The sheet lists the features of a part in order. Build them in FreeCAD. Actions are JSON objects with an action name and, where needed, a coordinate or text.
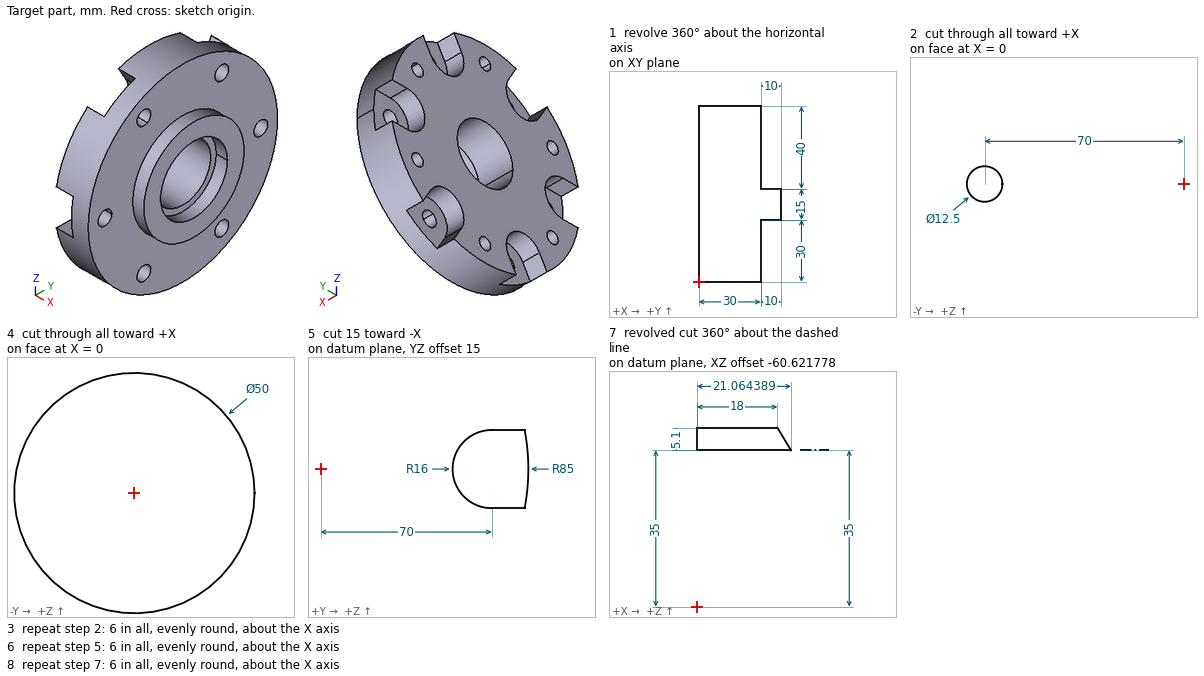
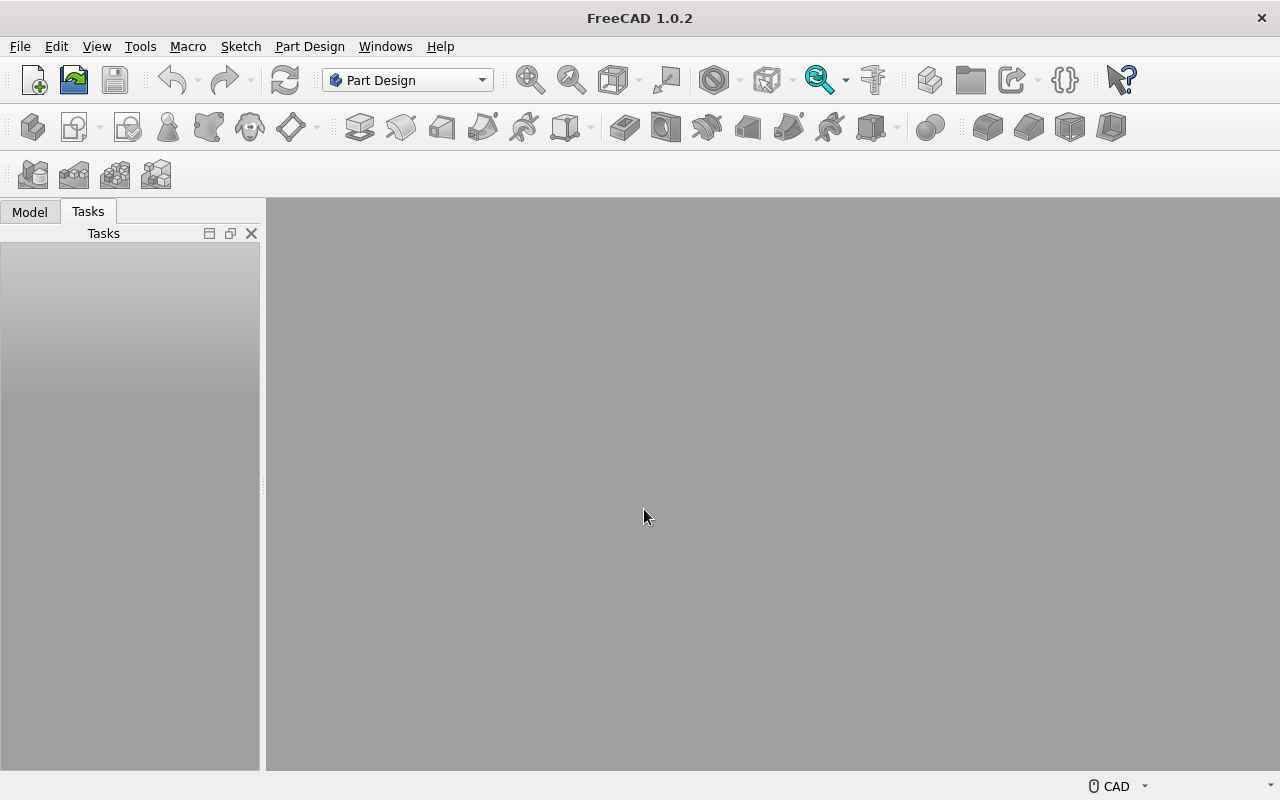
{"action": "left_click", "coordinate": [33, 80]}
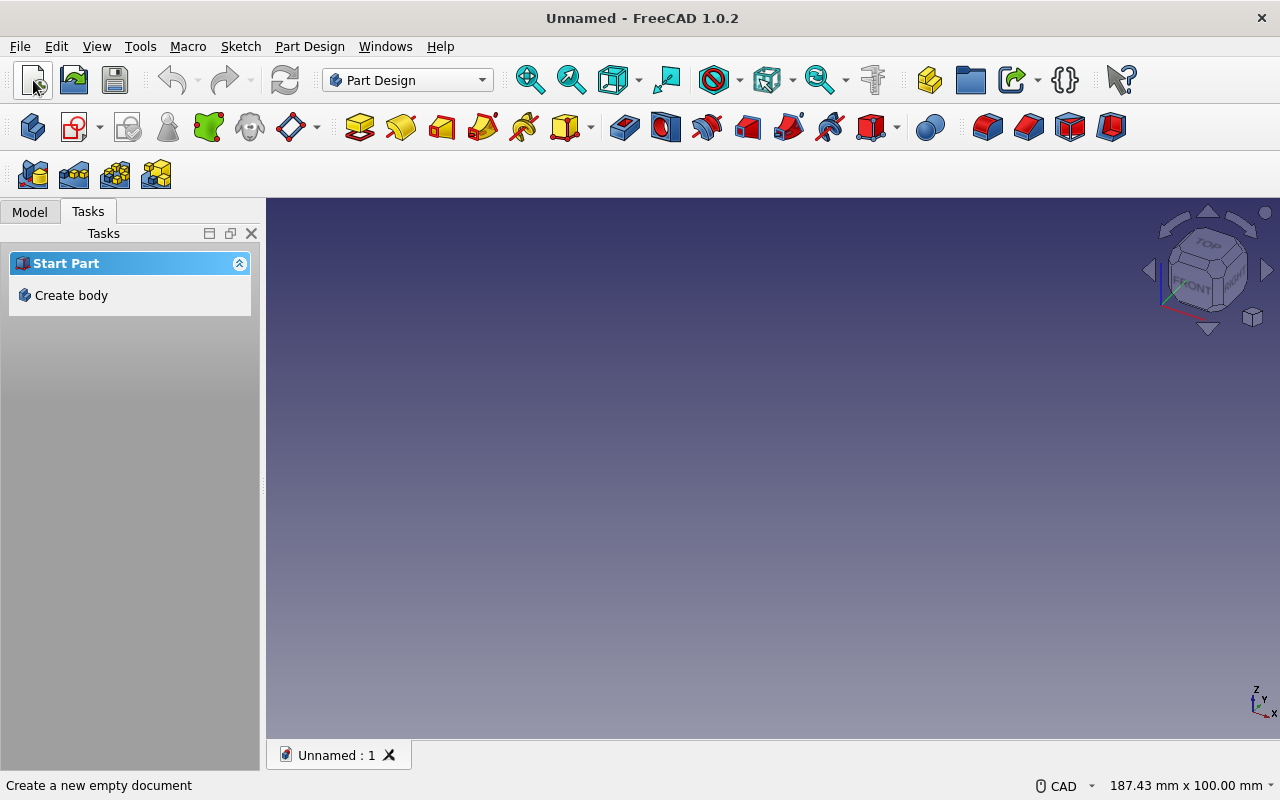
{"action": "left_click", "coordinate": [74, 128]}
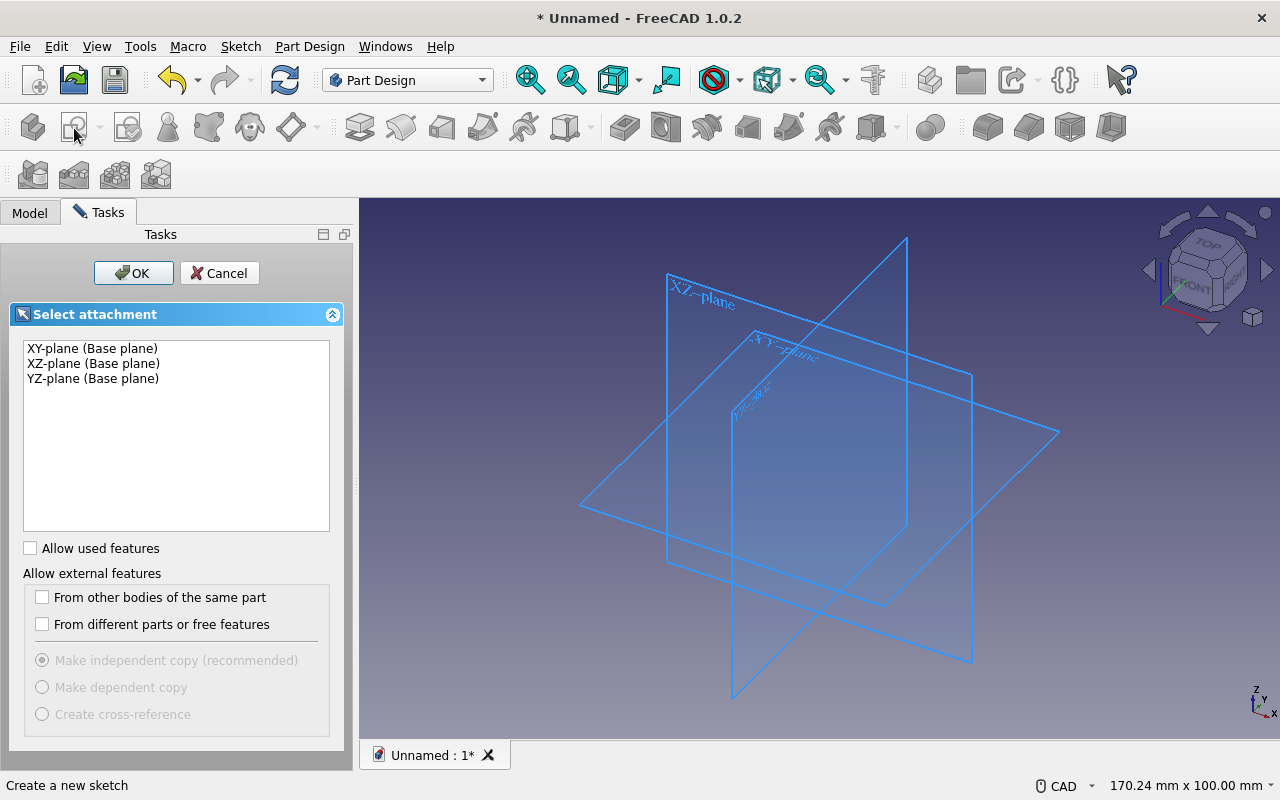
{"action": "left_click", "coordinate": [84, 348]}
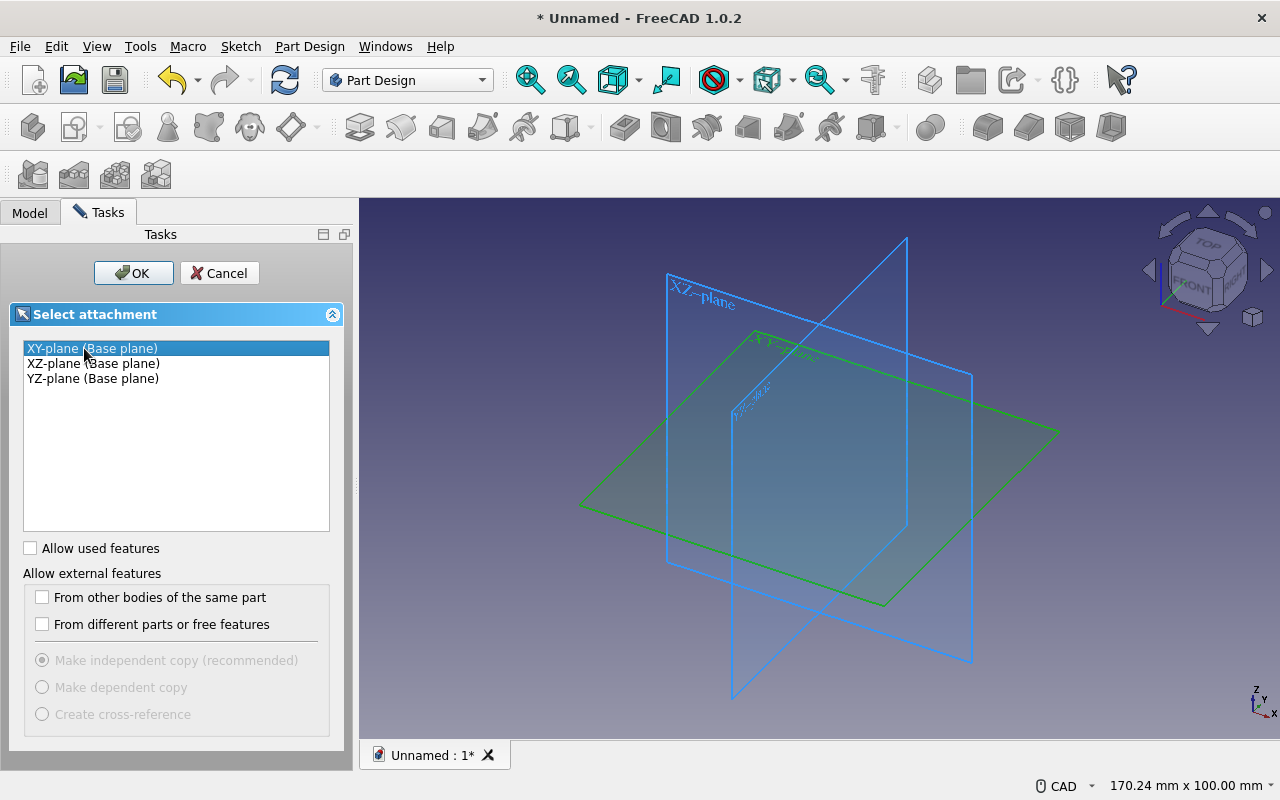
{"action": "left_click", "coordinate": [134, 273]}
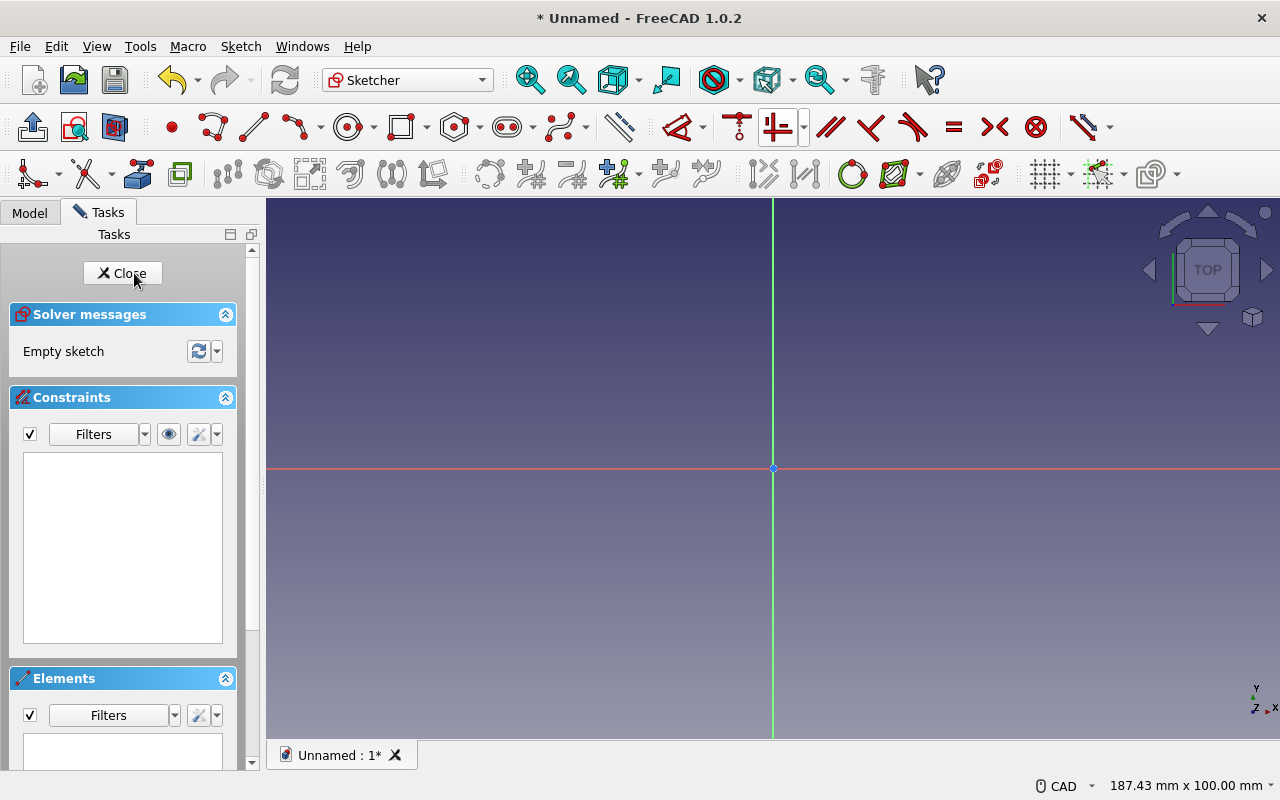
{"action": "scroll", "coordinate": [490, 711], "scroll_direction": "down", "scroll_amount": 3}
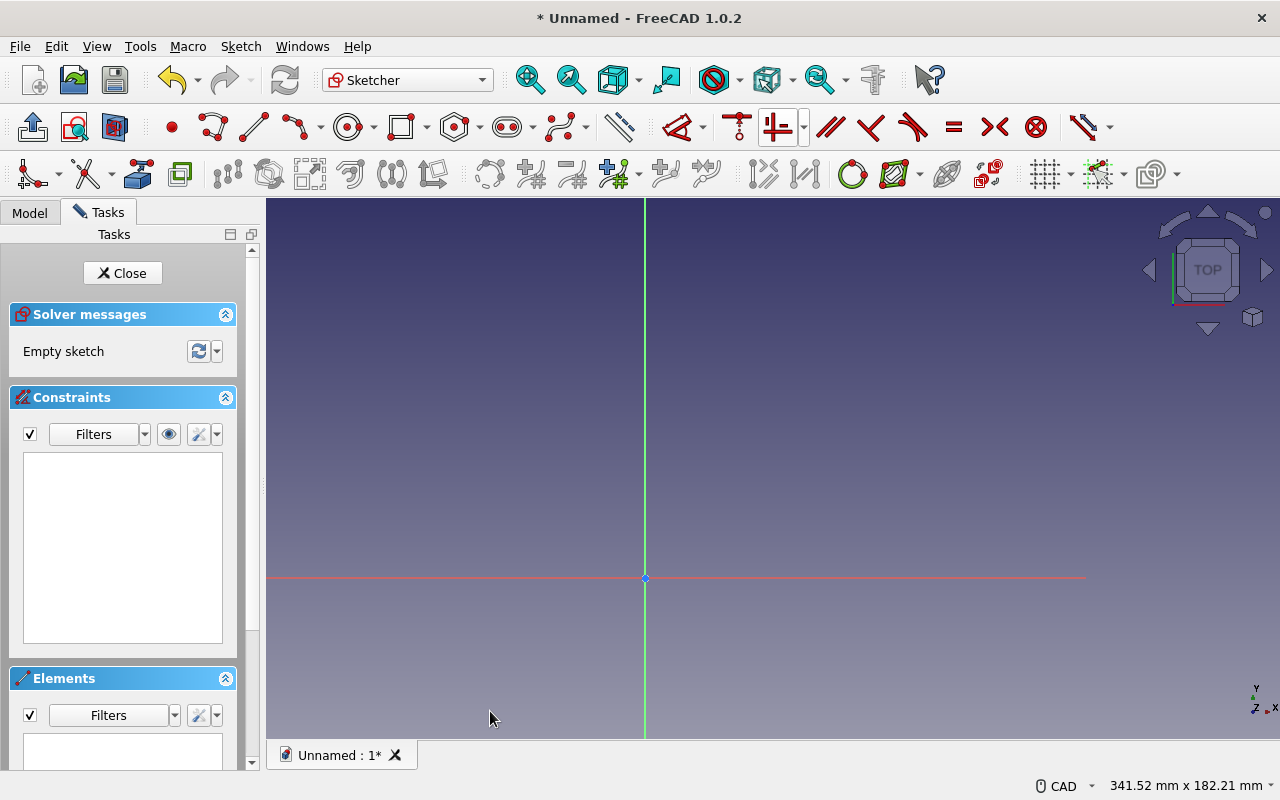
{"action": "scroll", "coordinate": [705, 419], "scroll_direction": "up", "scroll_amount": 2}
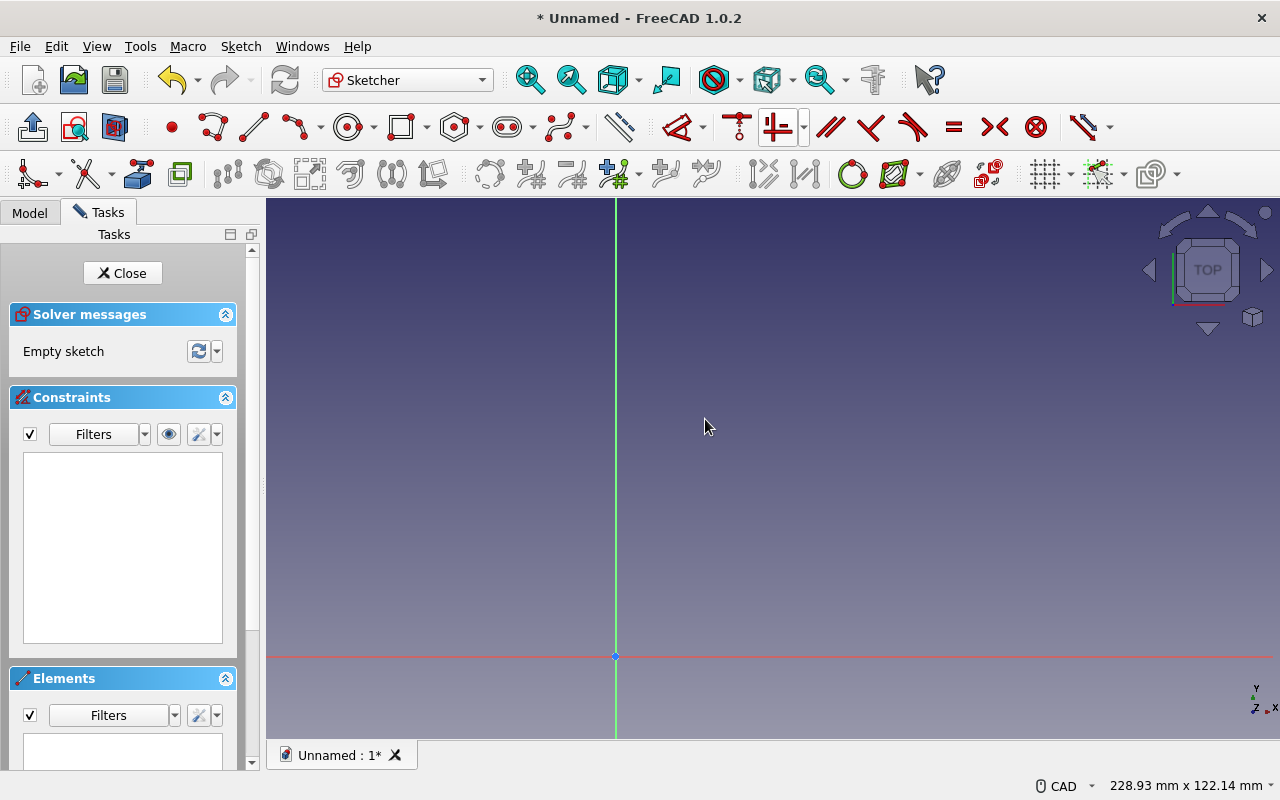
{"action": "left_click", "coordinate": [213, 128]}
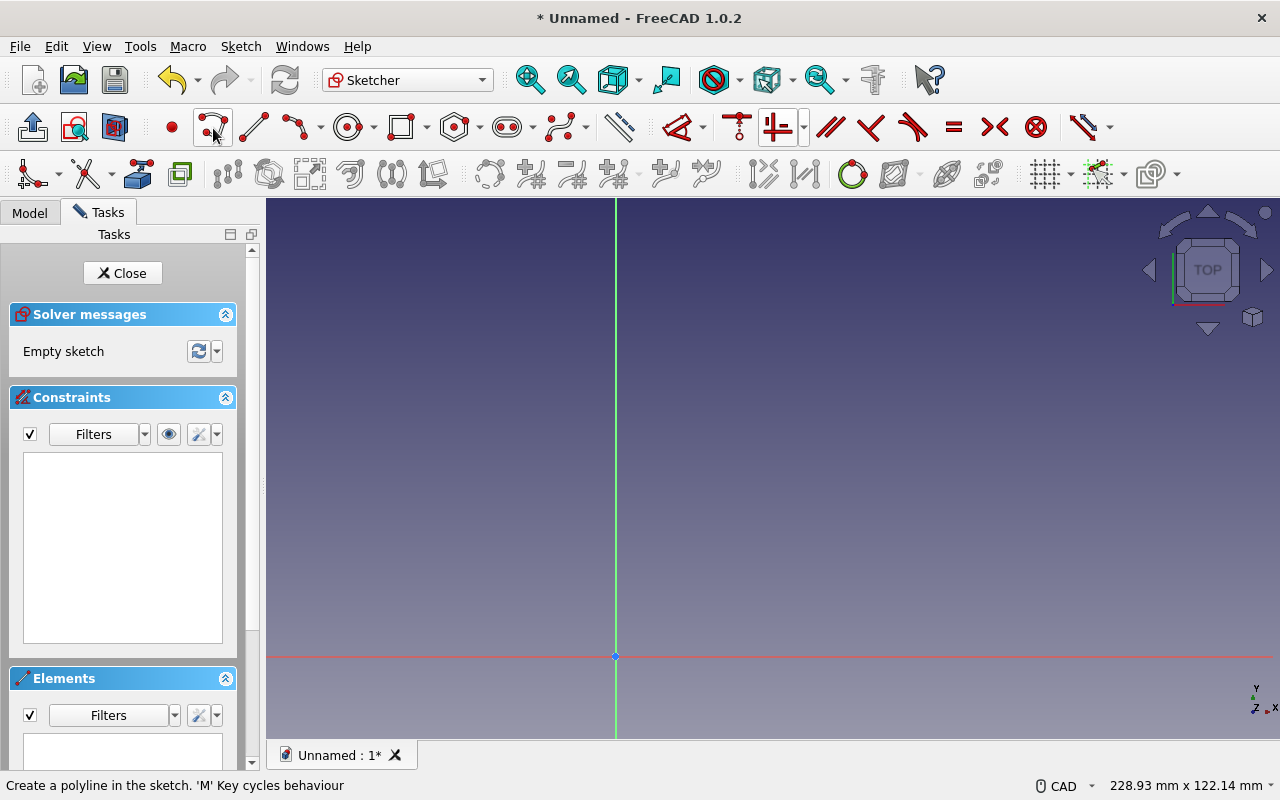
{"action": "left_click", "coordinate": [616, 657]}
{"action": "left_click", "coordinate": [749, 648]}
{"action": "left_click", "coordinate": [749, 524]}
{"action": "left_click", "coordinate": [793, 524]}
{"action": "left_click", "coordinate": [793, 457]}
{"action": "left_click", "coordinate": [749, 457]}
{"action": "left_click", "coordinate": [749, 280]}
{"action": "left_click", "coordinate": [625, 280]}
{"action": "left_click", "coordinate": [616, 657]}
{"action": "key", "text": "Escape"}
{"action": "key", "text": "Escape"}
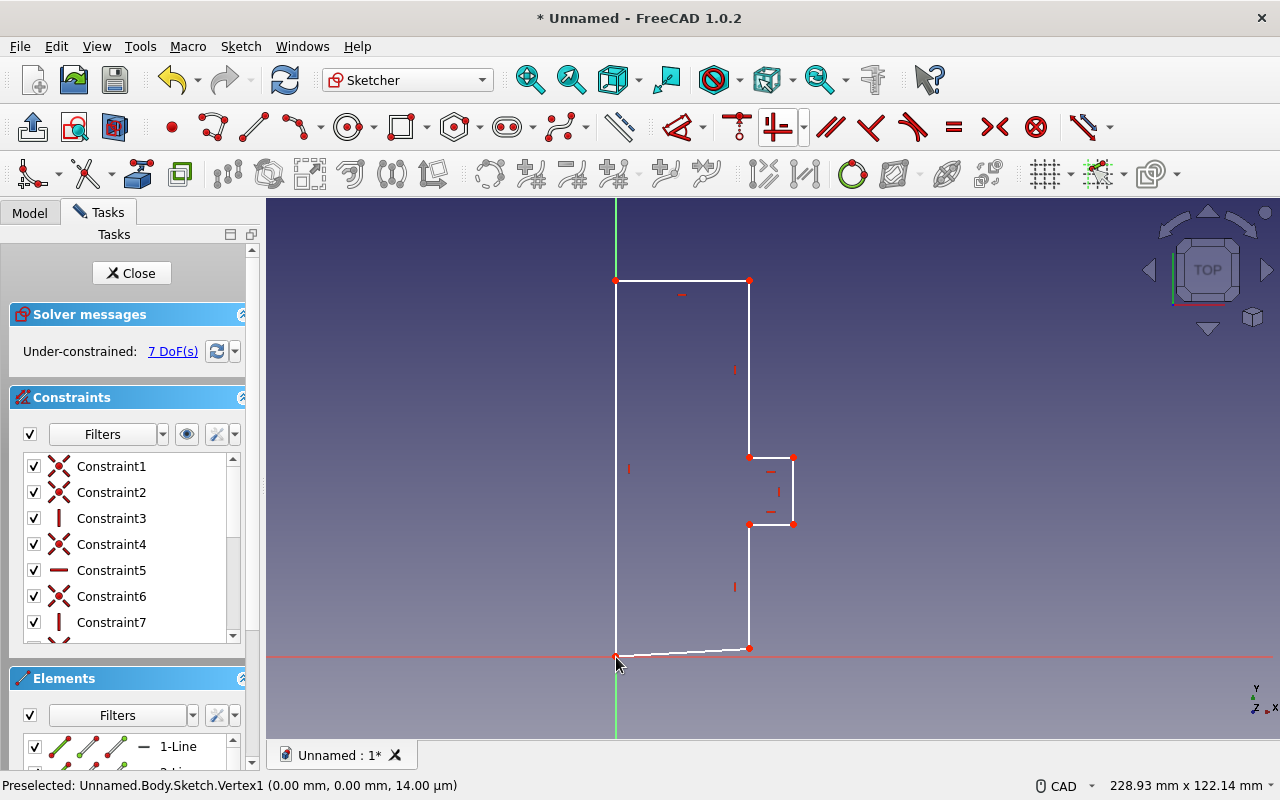
{"action": "left_click", "coordinate": [656, 654]}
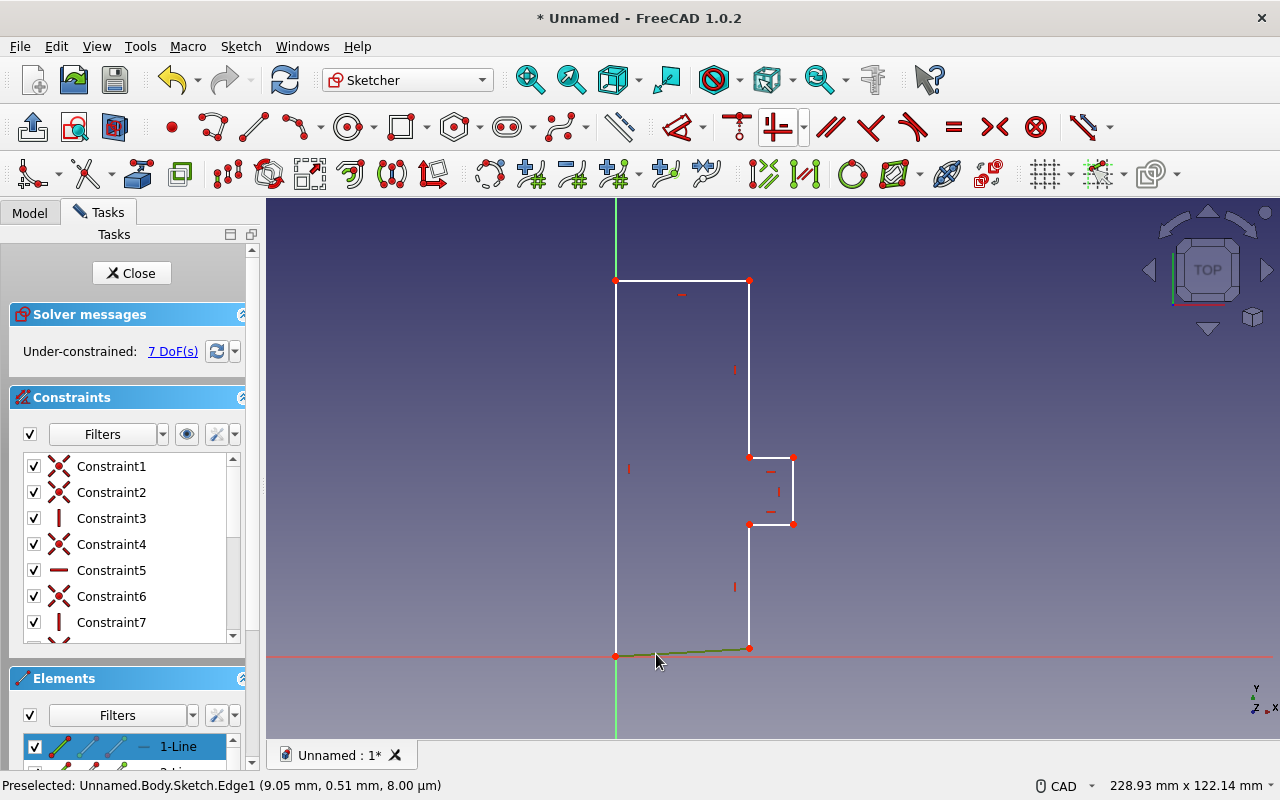
{"action": "left_click", "coordinate": [804, 128]}